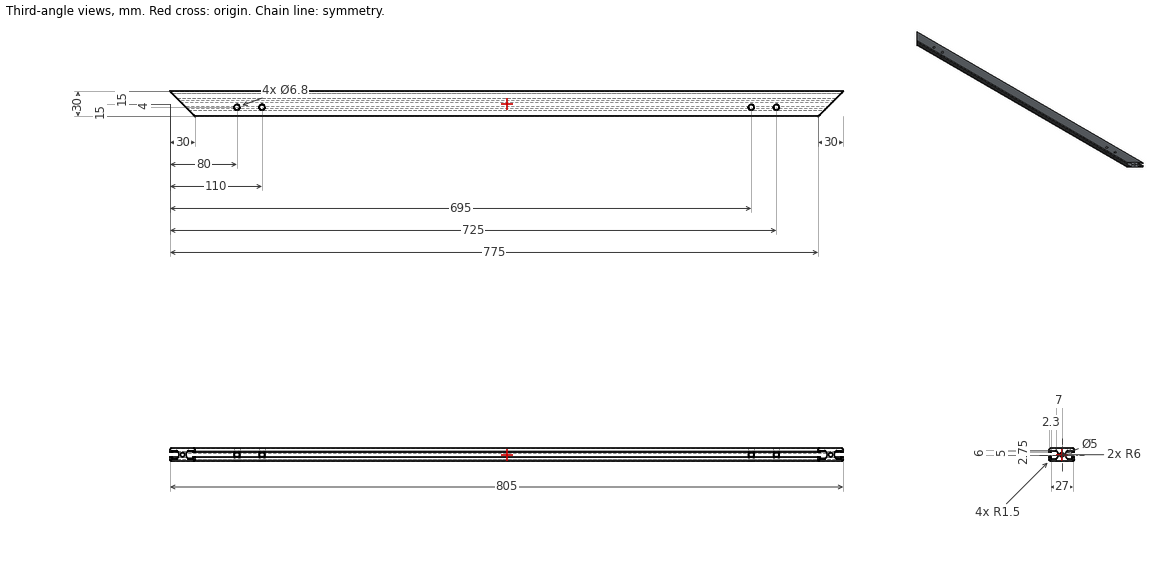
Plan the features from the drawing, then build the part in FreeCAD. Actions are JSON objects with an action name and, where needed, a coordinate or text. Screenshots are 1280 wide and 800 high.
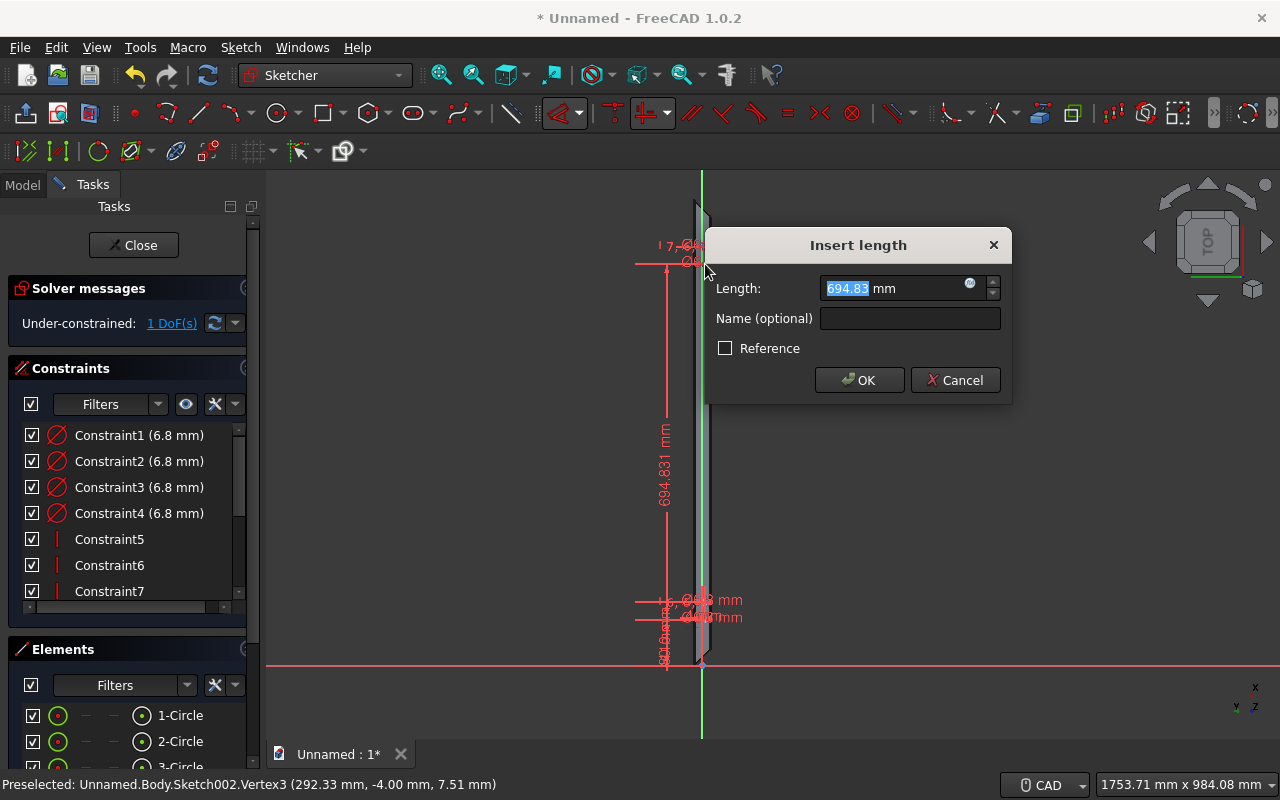
{"action": "type", "text": "695"}
{"action": "key", "text": "Return"}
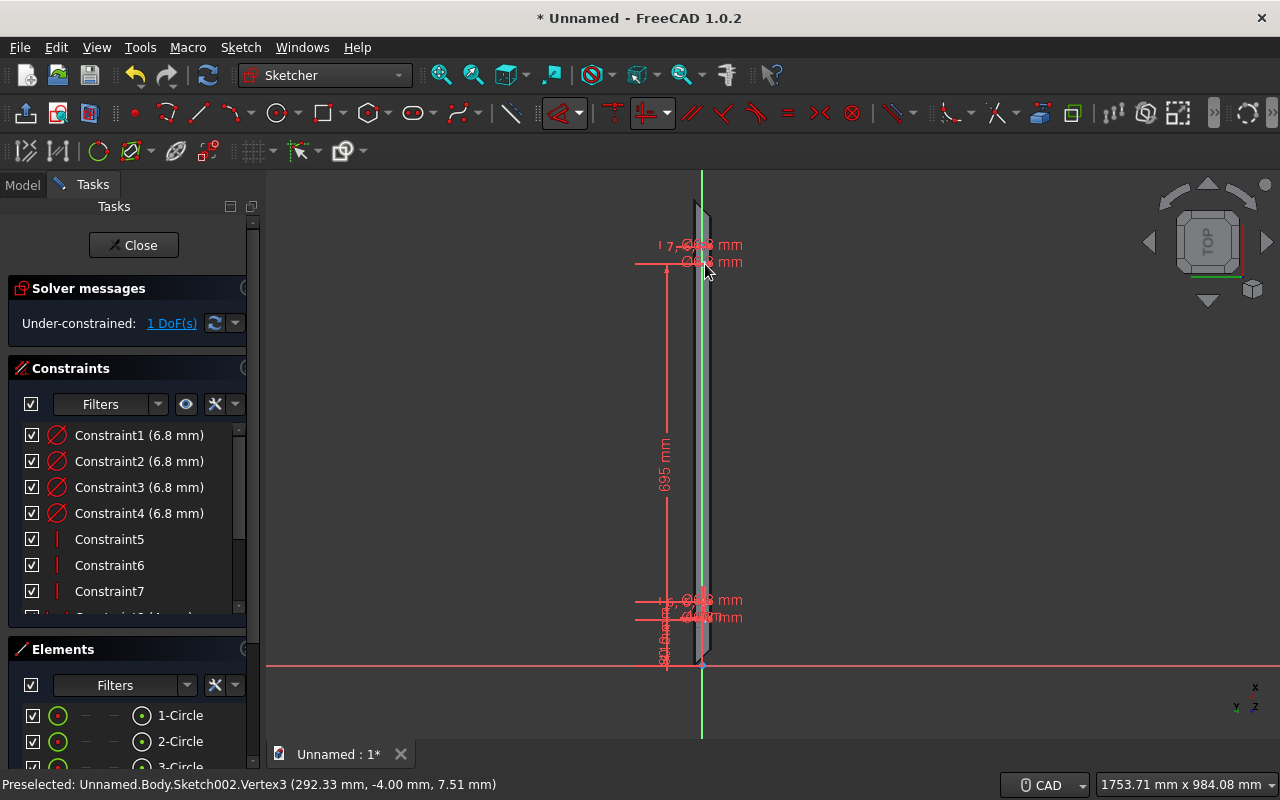
{"action": "scroll", "coordinate": [705, 247], "scroll_direction": "up", "scroll_amount": 4}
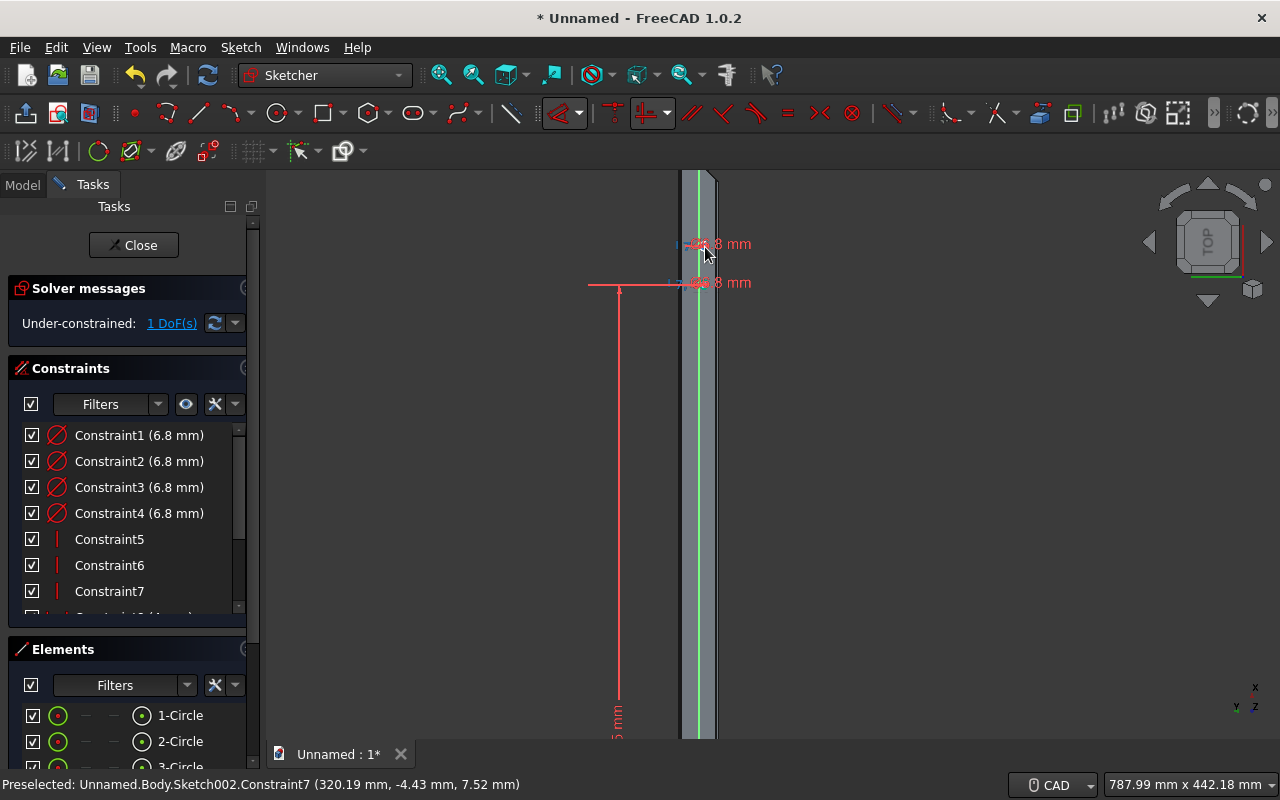
{"action": "left_click", "coordinate": [704, 246]}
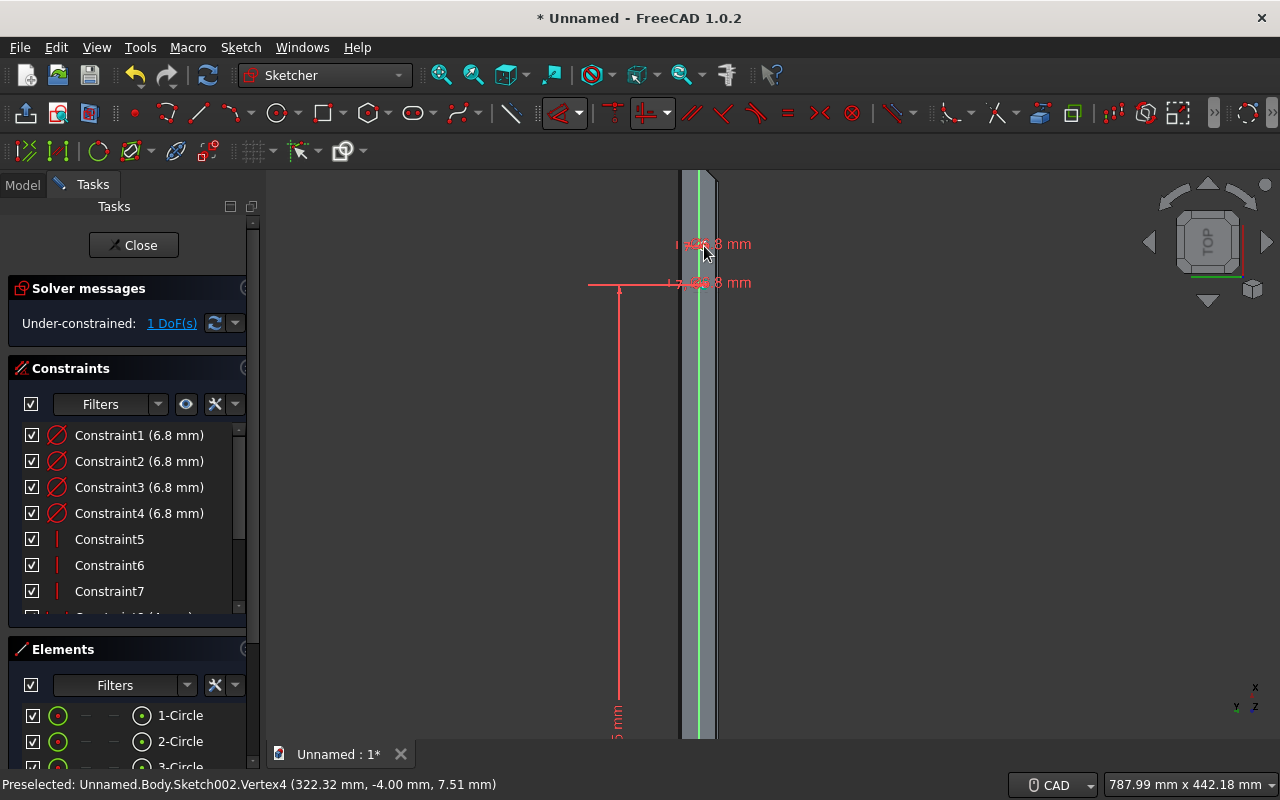
{"action": "left_click", "coordinate": [582, 114]}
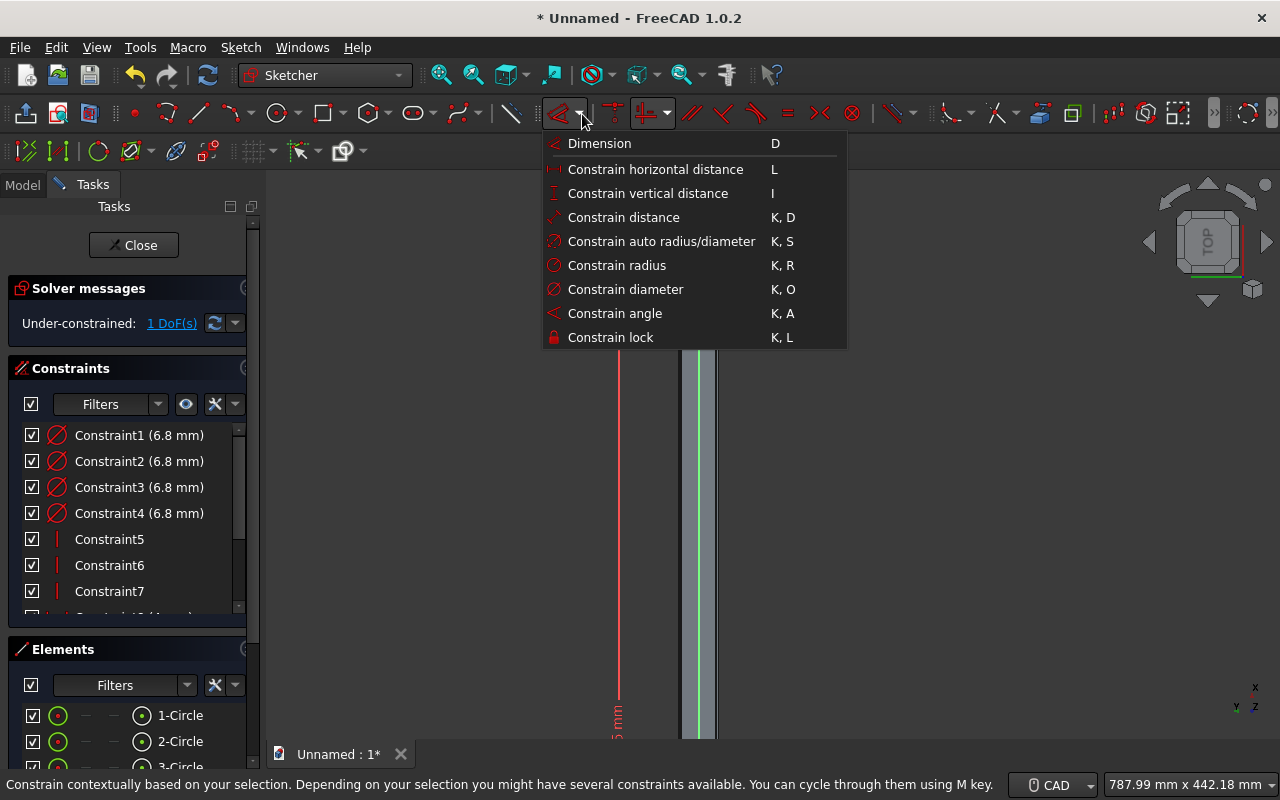
{"action": "left_click", "coordinate": [695, 193]}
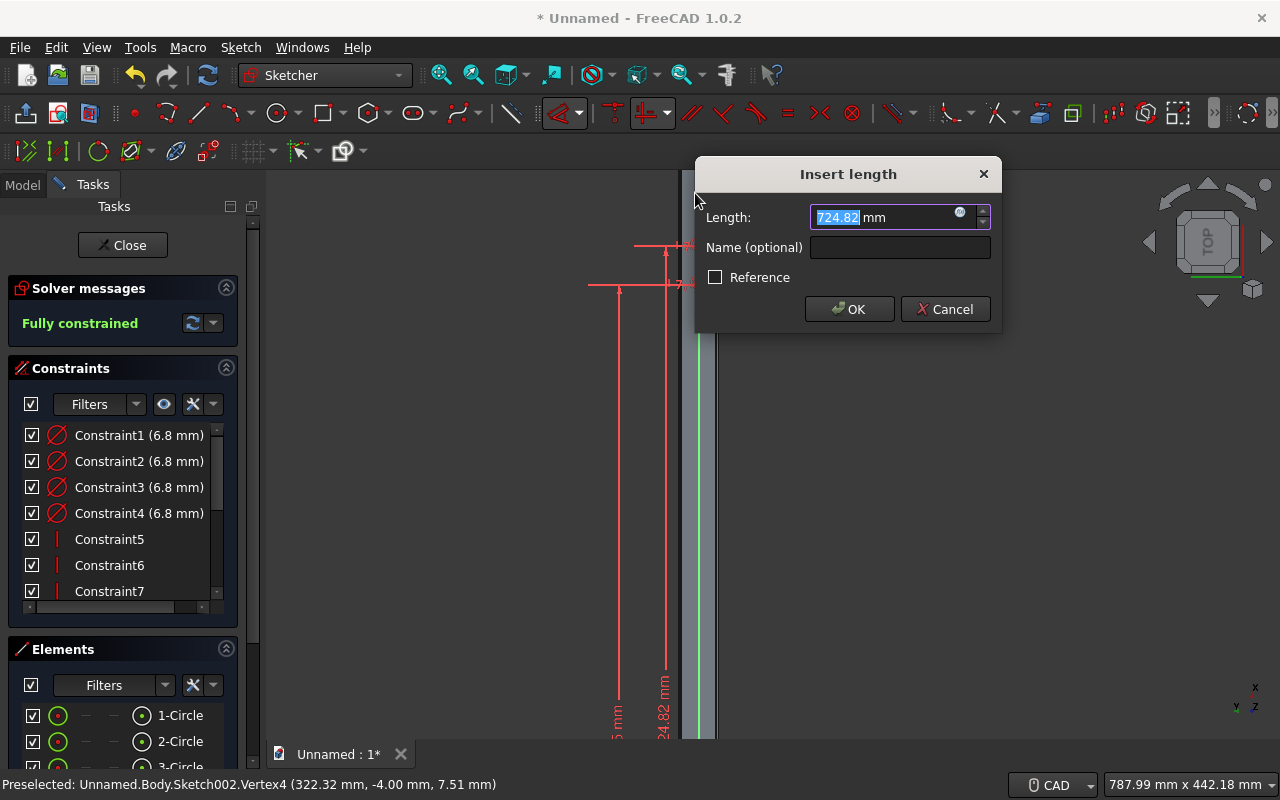
{"action": "type", "text": "725"}
{"action": "key", "text": "Return"}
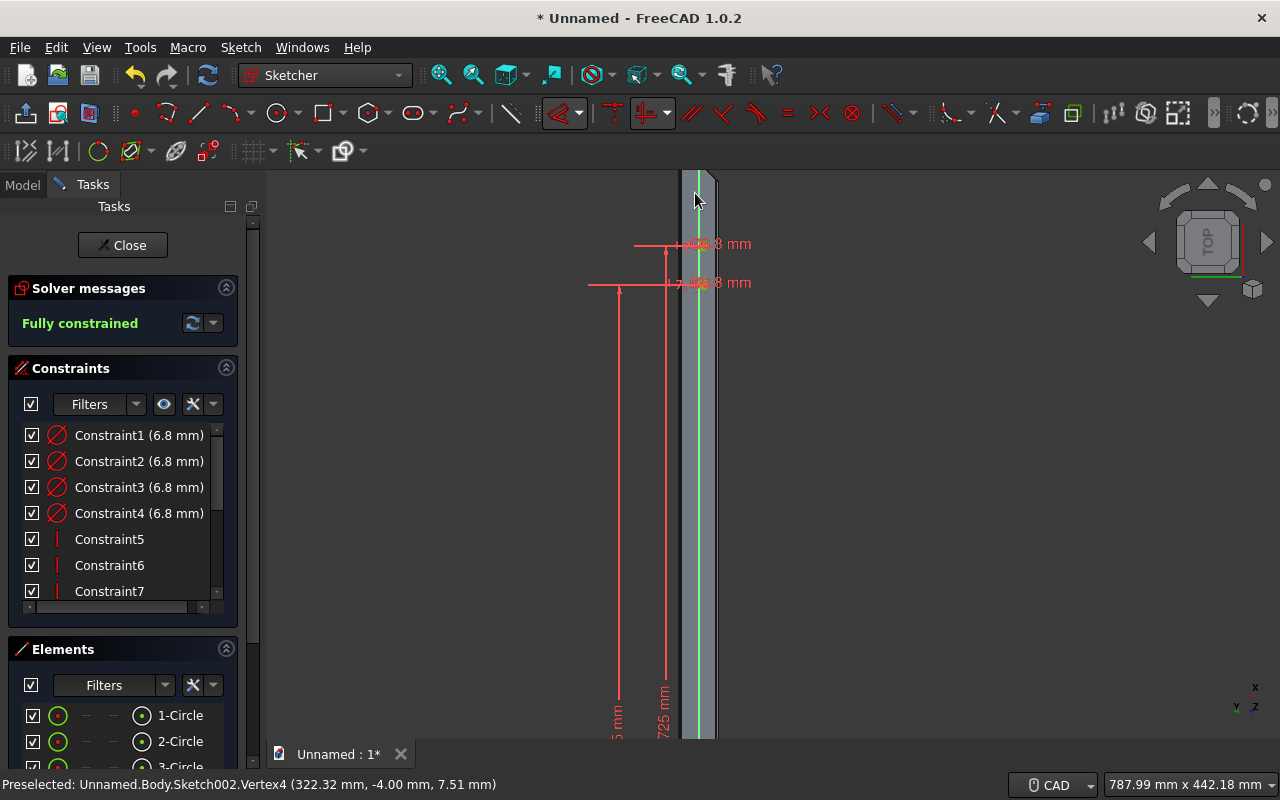
{"action": "left_click", "coordinate": [123, 245]}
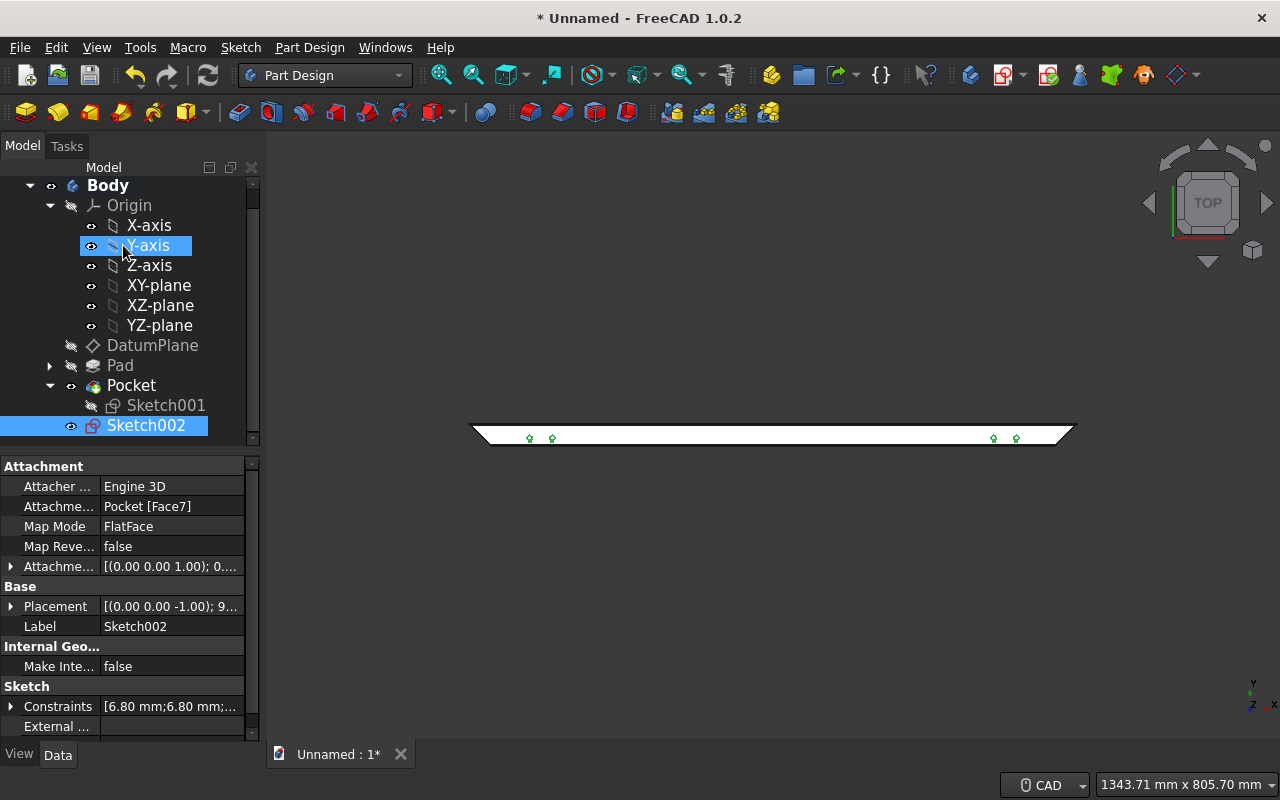
{"action": "left_click", "coordinate": [240, 112]}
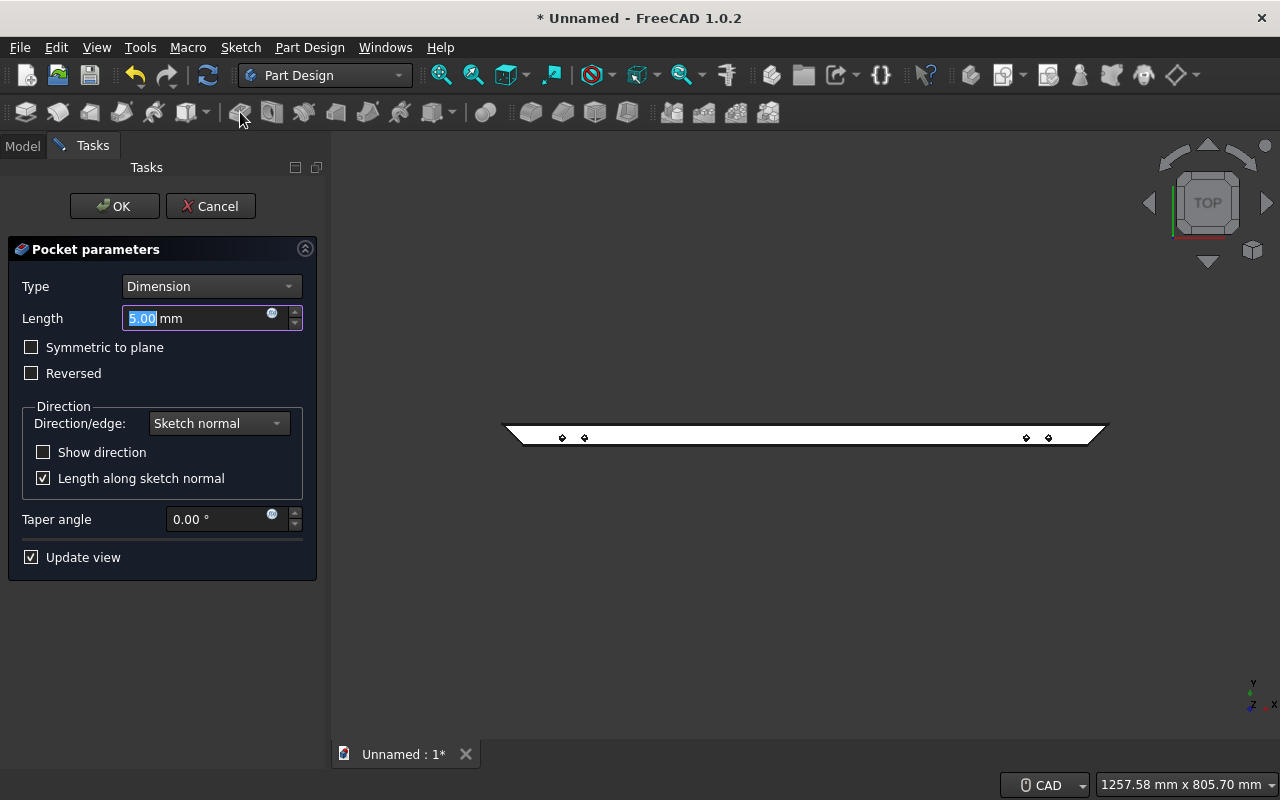
{"action": "left_click", "coordinate": [212, 286]}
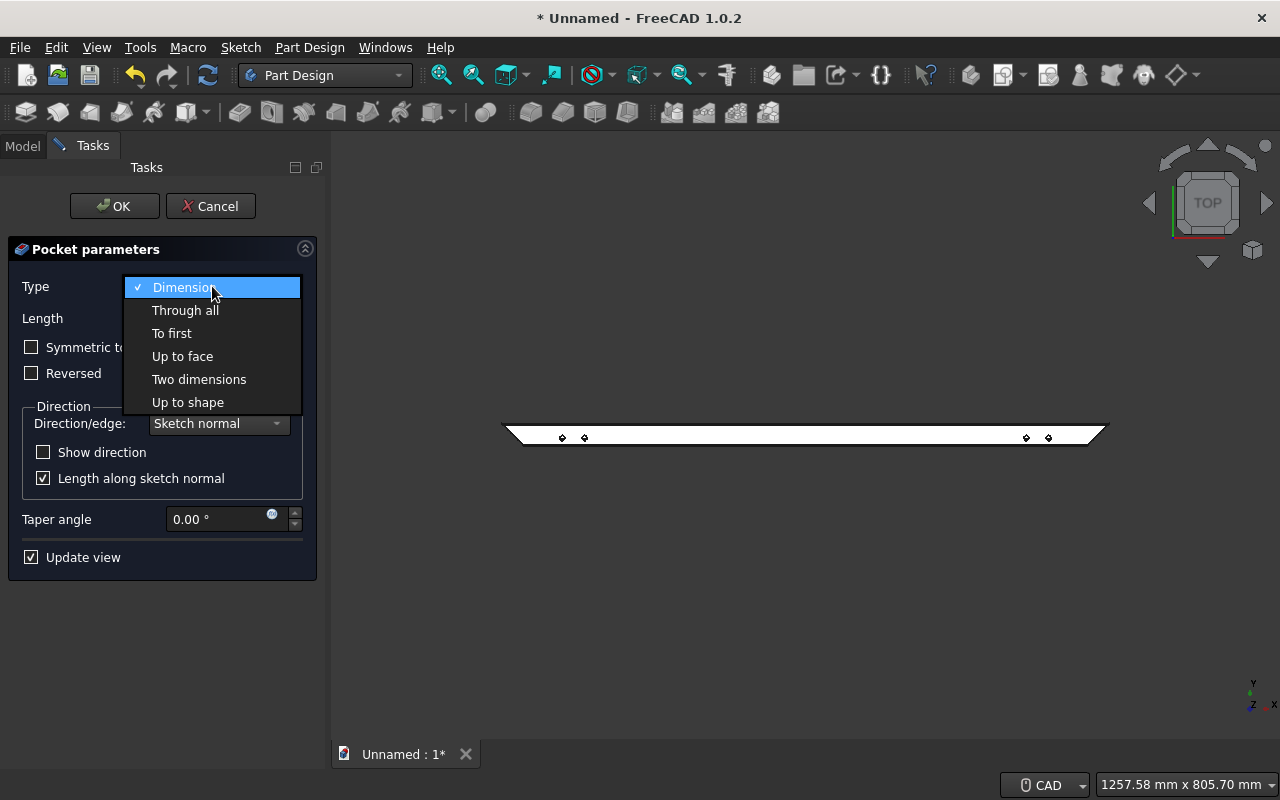
{"action": "left_click", "coordinate": [212, 310]}